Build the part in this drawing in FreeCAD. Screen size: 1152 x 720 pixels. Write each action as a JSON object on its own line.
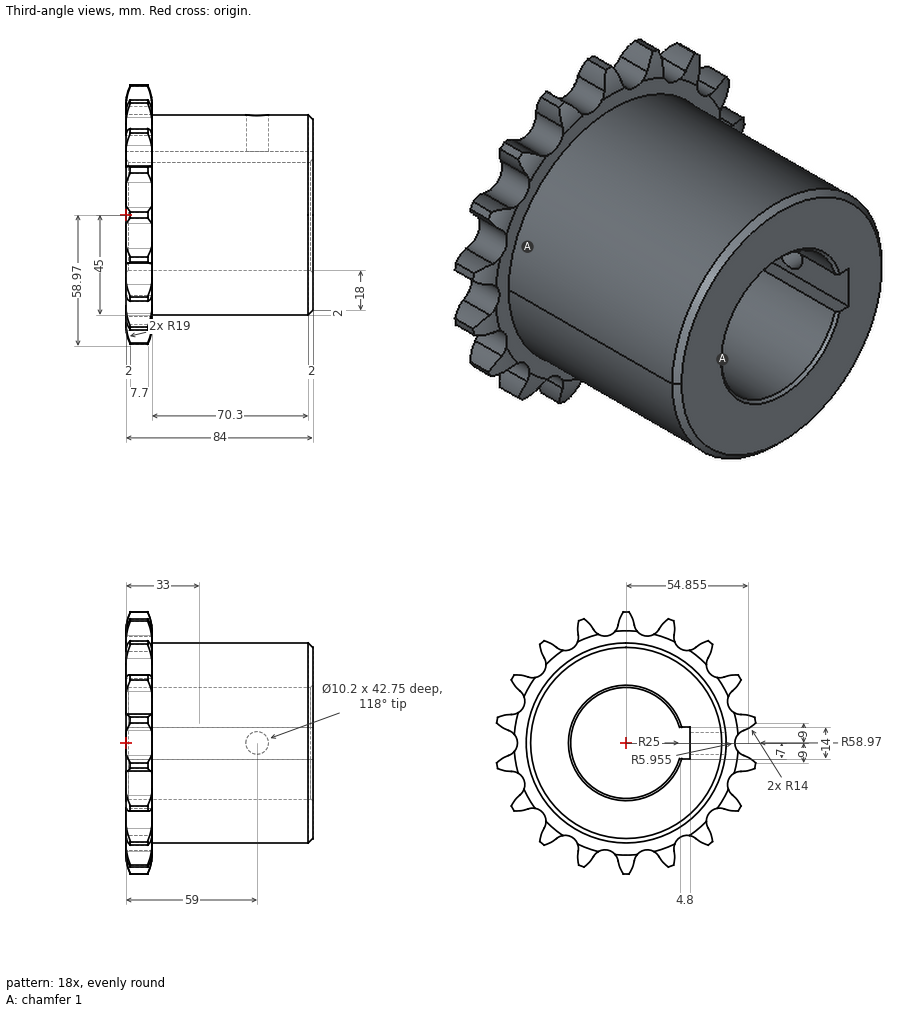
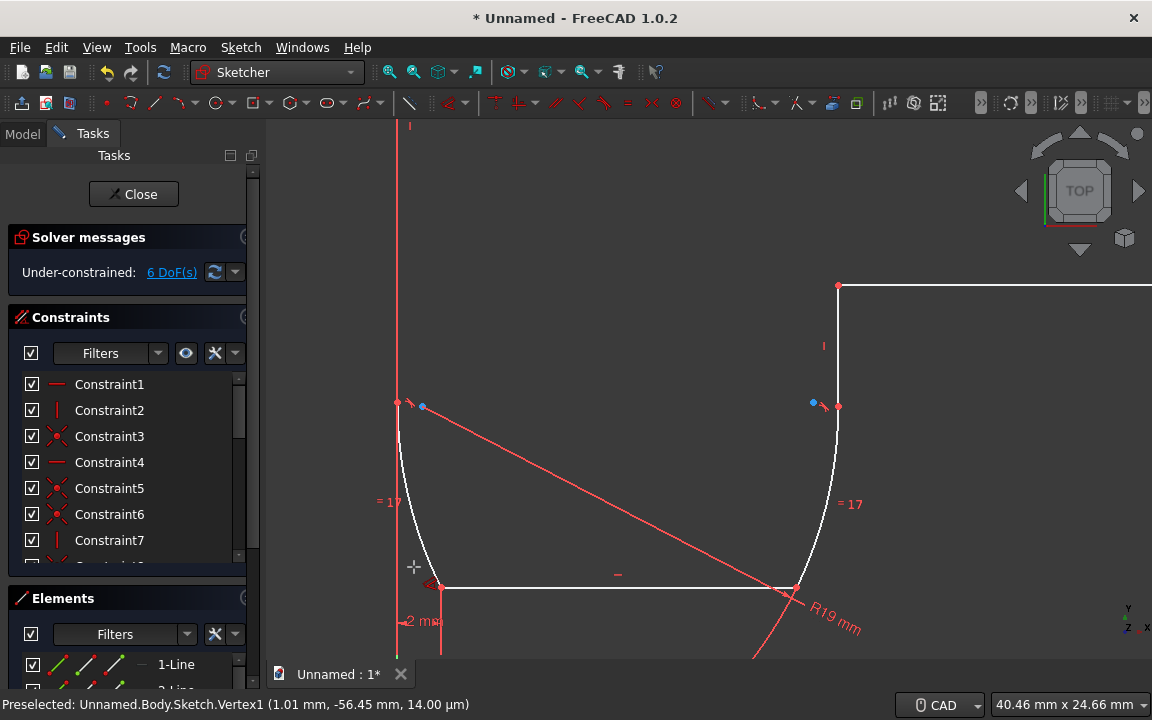
{"action": "scroll", "coordinate": [419, 535], "scroll_direction": "down", "scroll_amount": 7}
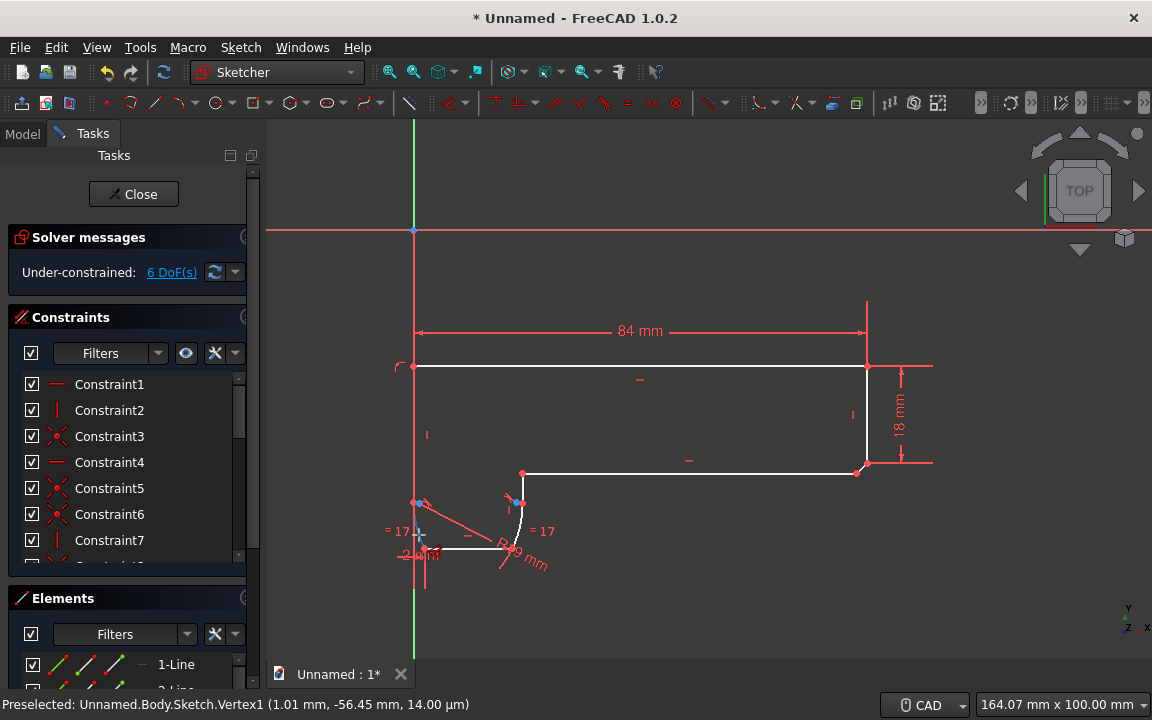
{"action": "scroll", "coordinate": [860, 471], "scroll_direction": "up", "scroll_amount": 7}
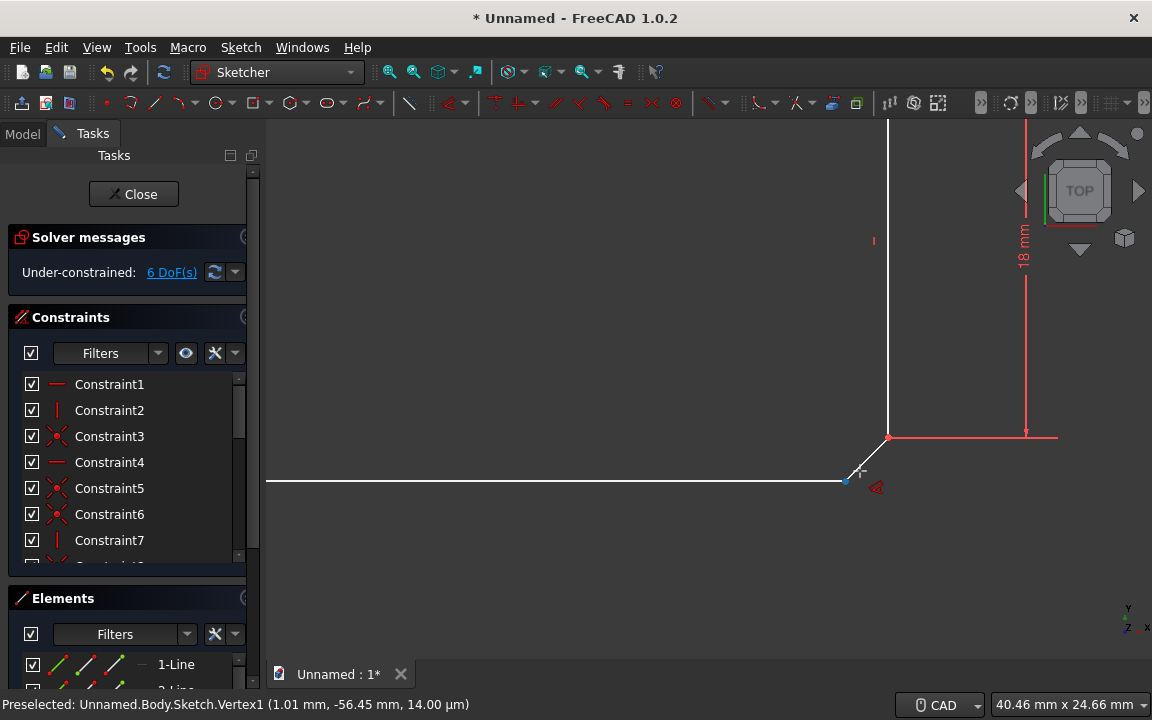
{"action": "left_click", "coordinate": [858, 468]}
{"action": "left_click", "coordinate": [867, 515]}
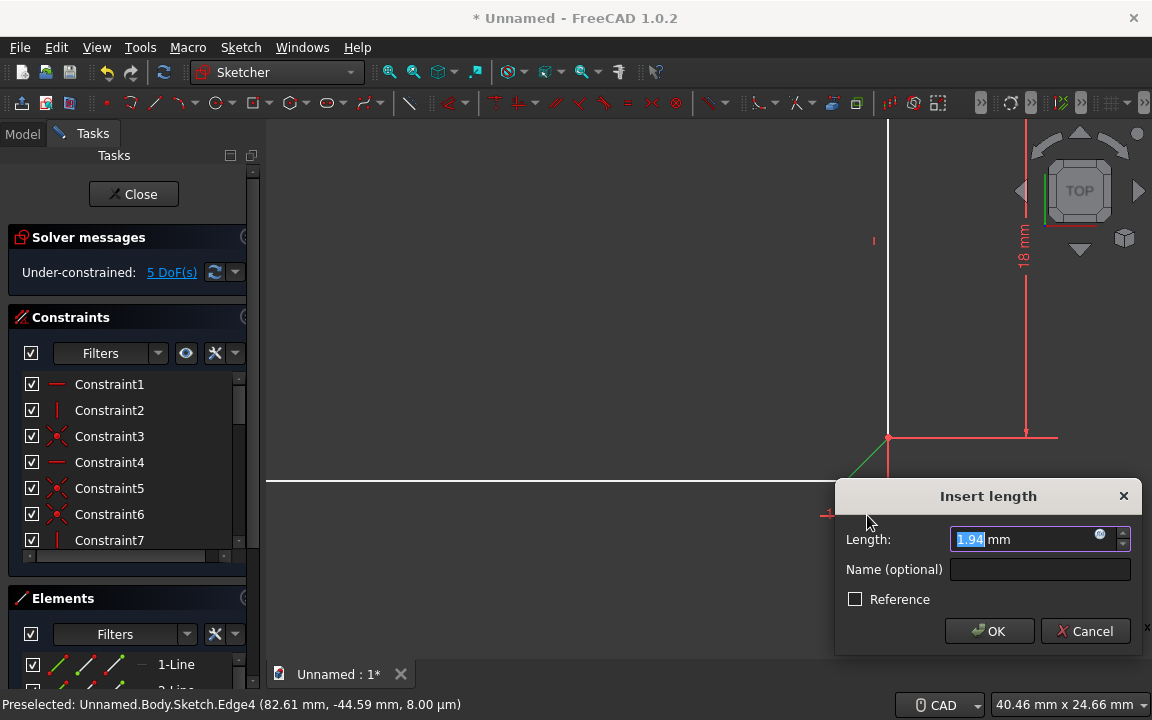
{"action": "type", "text": "2"}
{"action": "key", "text": "Return"}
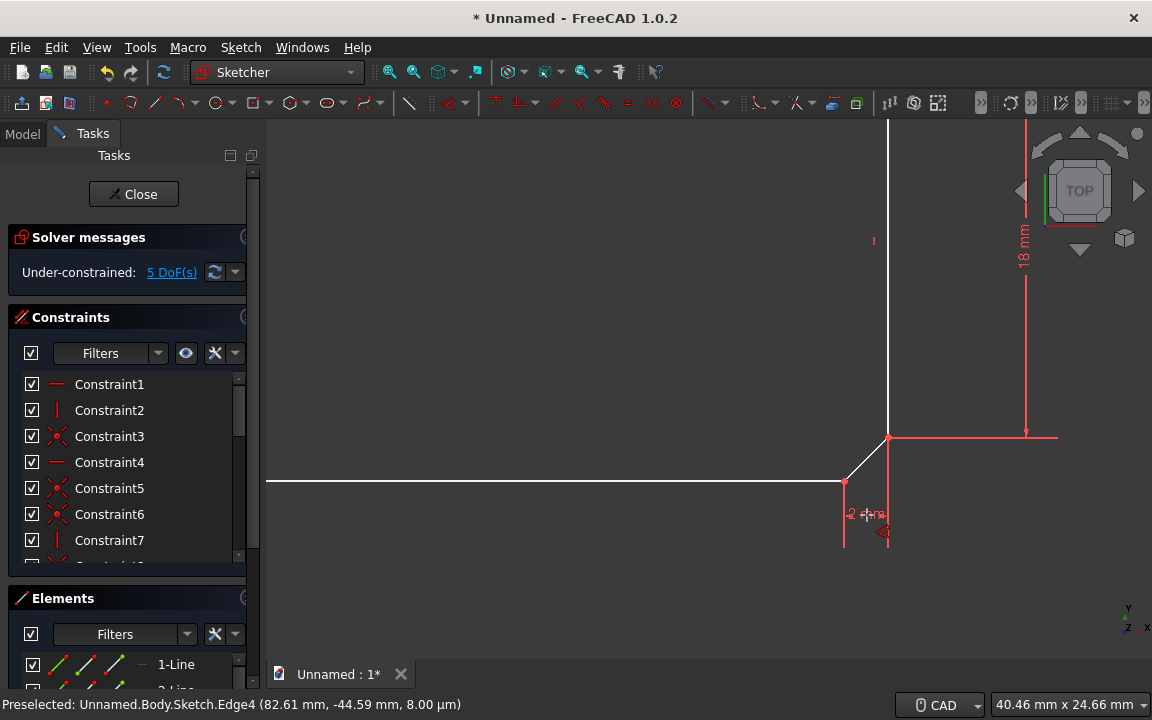
{"action": "left_click", "coordinate": [857, 468]}
{"action": "left_click", "coordinate": [922, 460]}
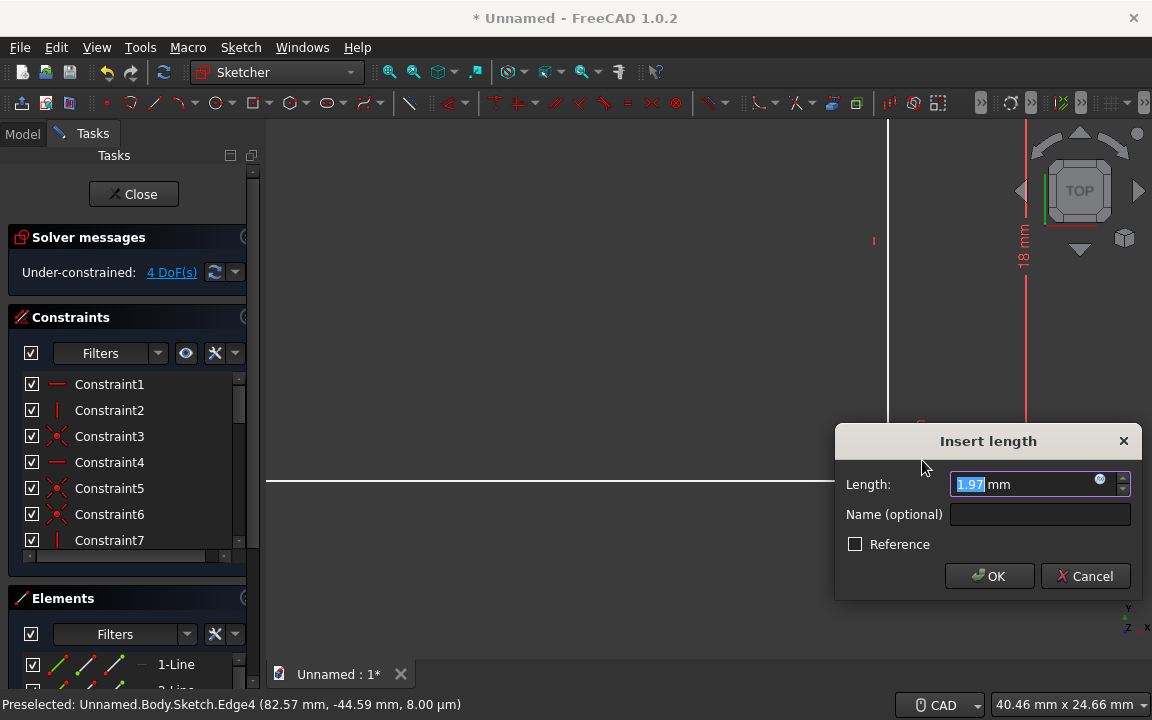
{"action": "type", "text": "2"}
{"action": "key", "text": "Return"}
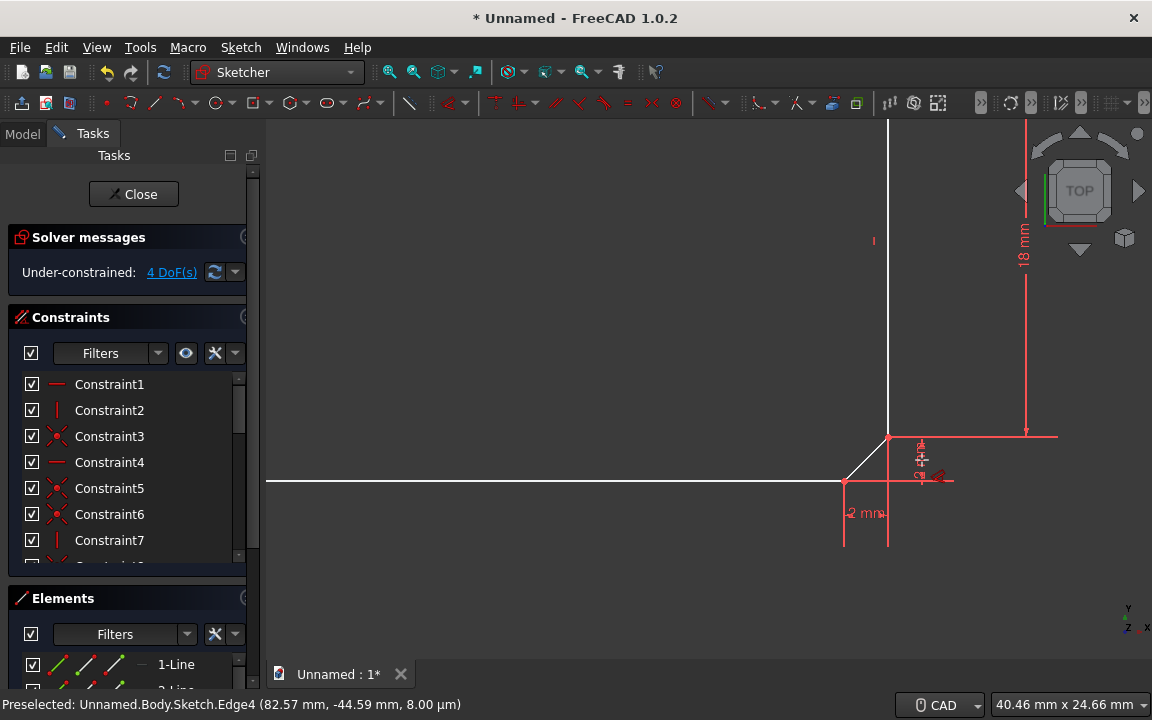
{"action": "scroll", "coordinate": [861, 471], "scroll_direction": "down", "scroll_amount": 7}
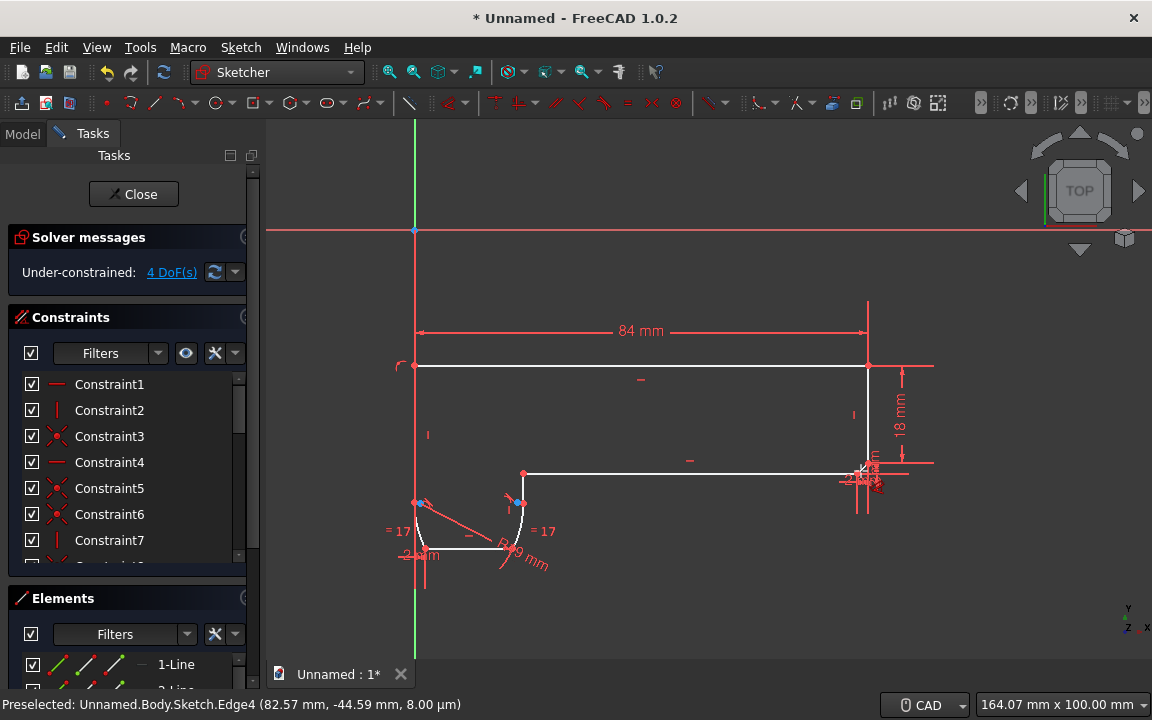
{"action": "left_click", "coordinate": [452, 549]}
{"action": "left_click", "coordinate": [469, 583]}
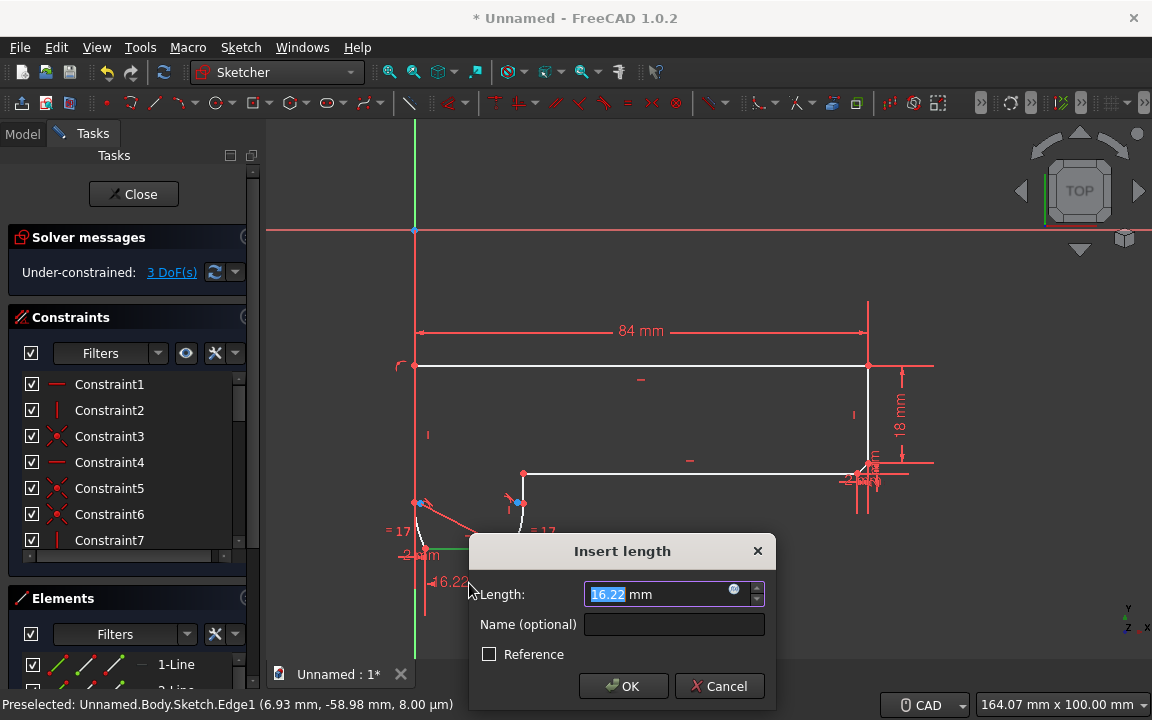
{"action": "type", "text": "7.7"}
{"action": "key", "text": "Return"}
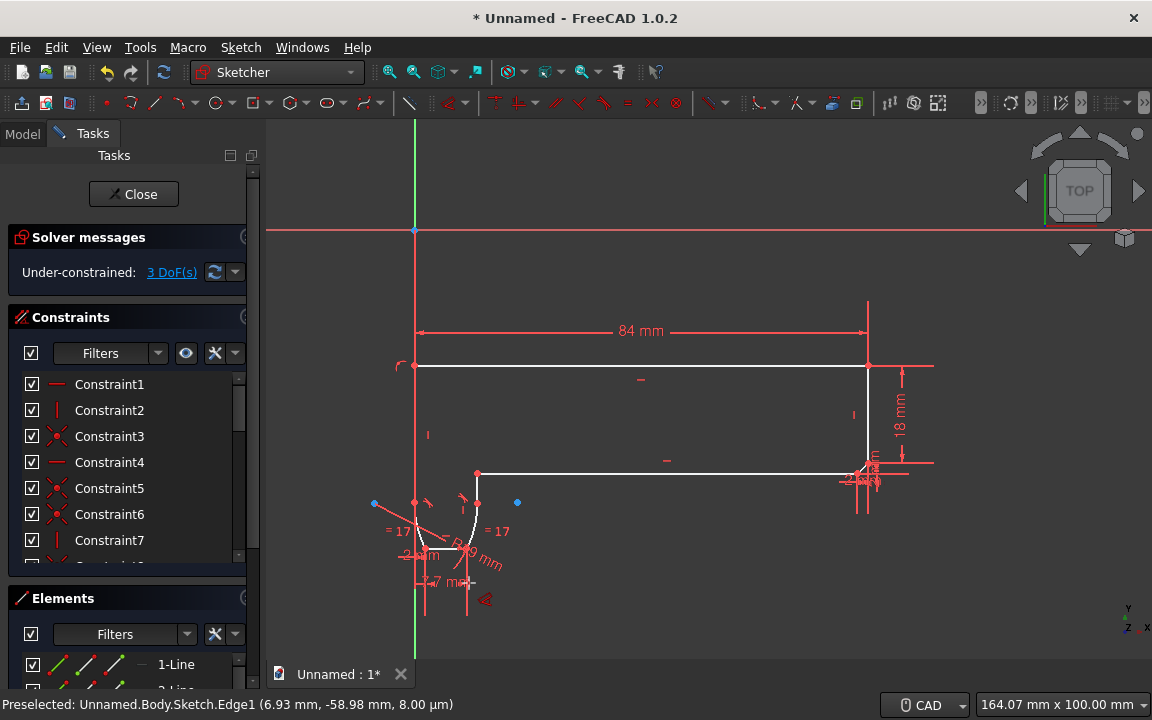
{"action": "left_click", "coordinate": [477, 474]}
{"action": "left_click", "coordinate": [381, 352]}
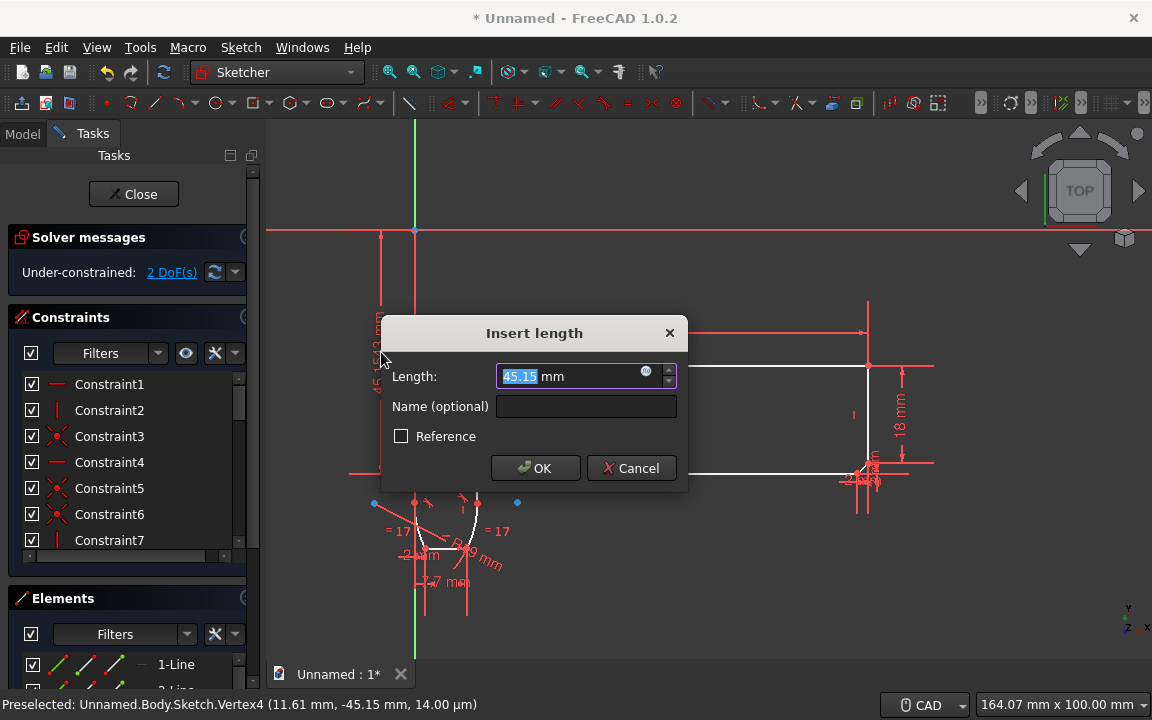
{"action": "type", "text": "45"}
{"action": "key", "text": "Return"}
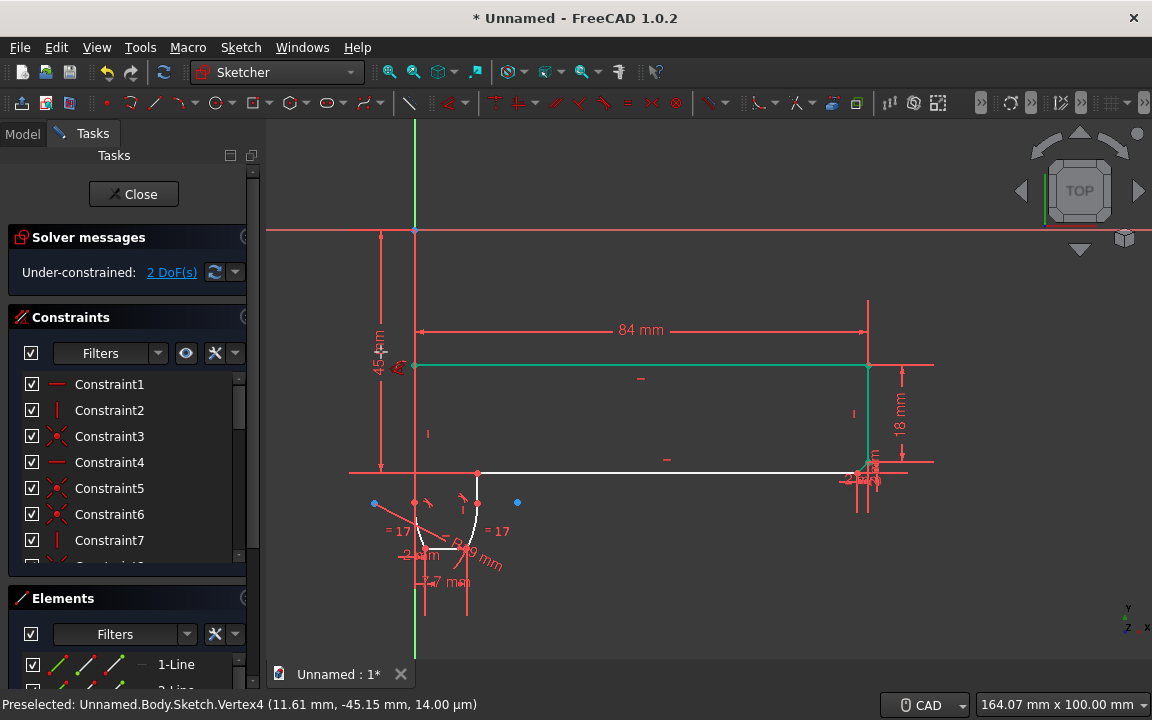
{"action": "left_click", "coordinate": [591, 473]}
{"action": "left_click", "coordinate": [667, 507]}